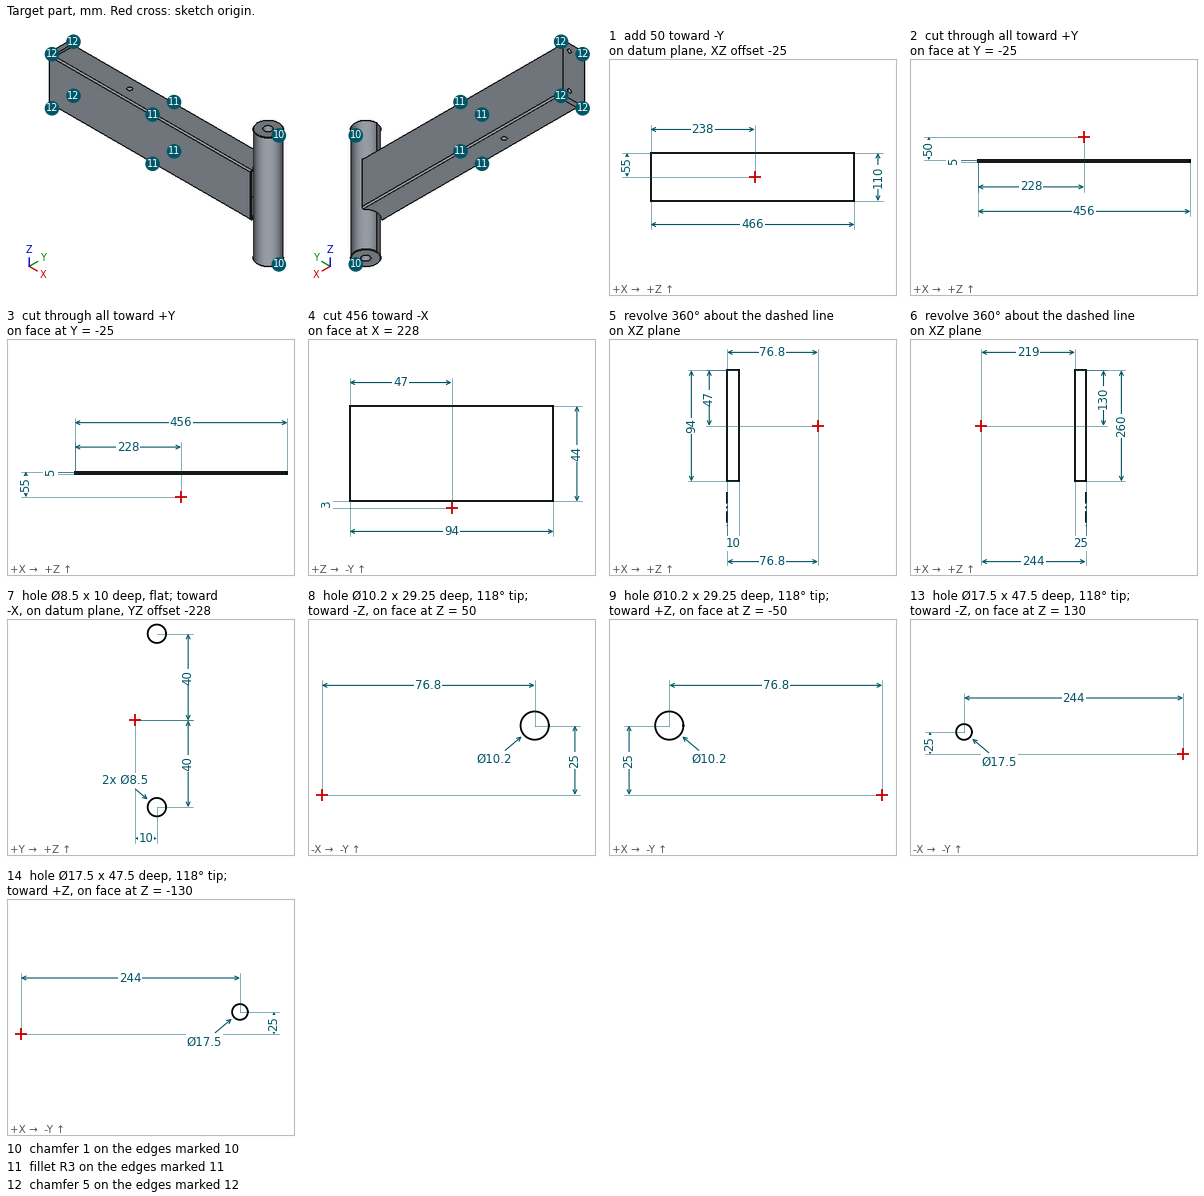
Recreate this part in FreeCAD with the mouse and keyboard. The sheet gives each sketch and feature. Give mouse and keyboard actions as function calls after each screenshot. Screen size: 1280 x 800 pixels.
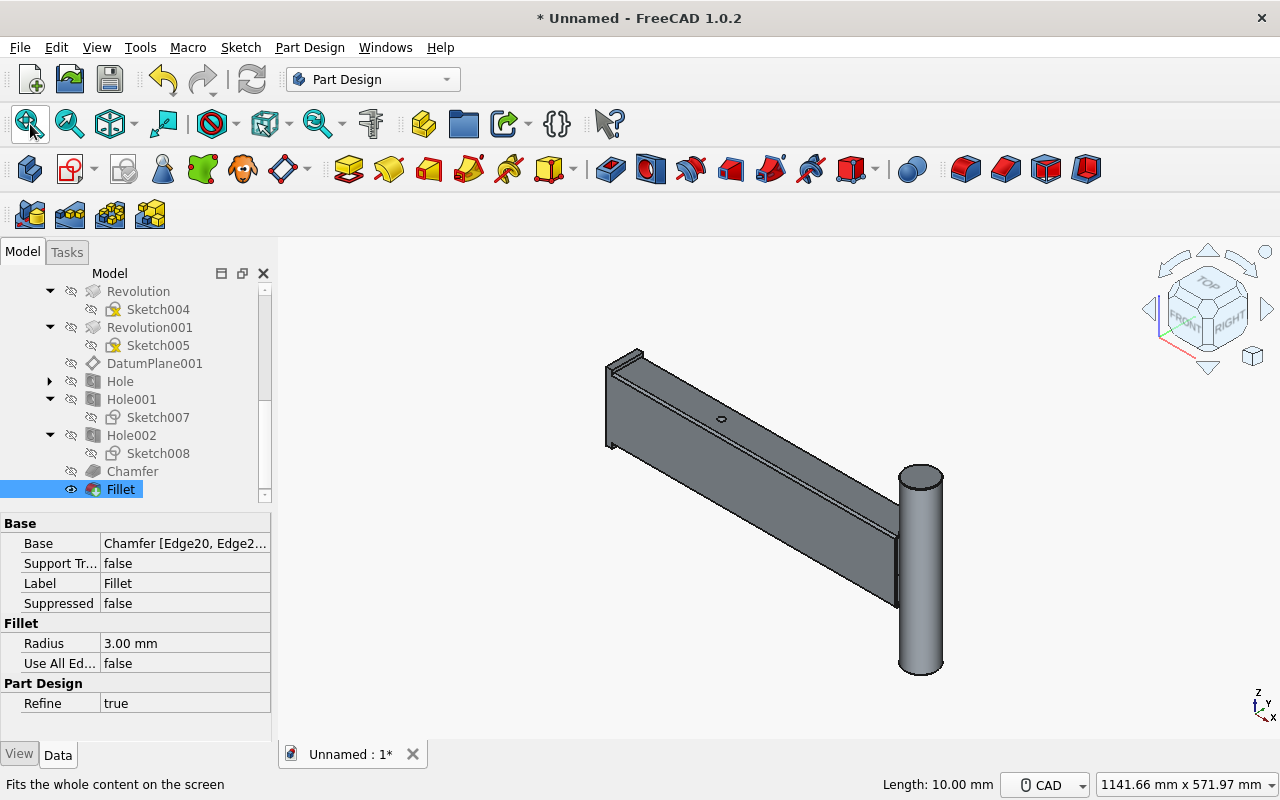
scroll(609, 446, up, 8)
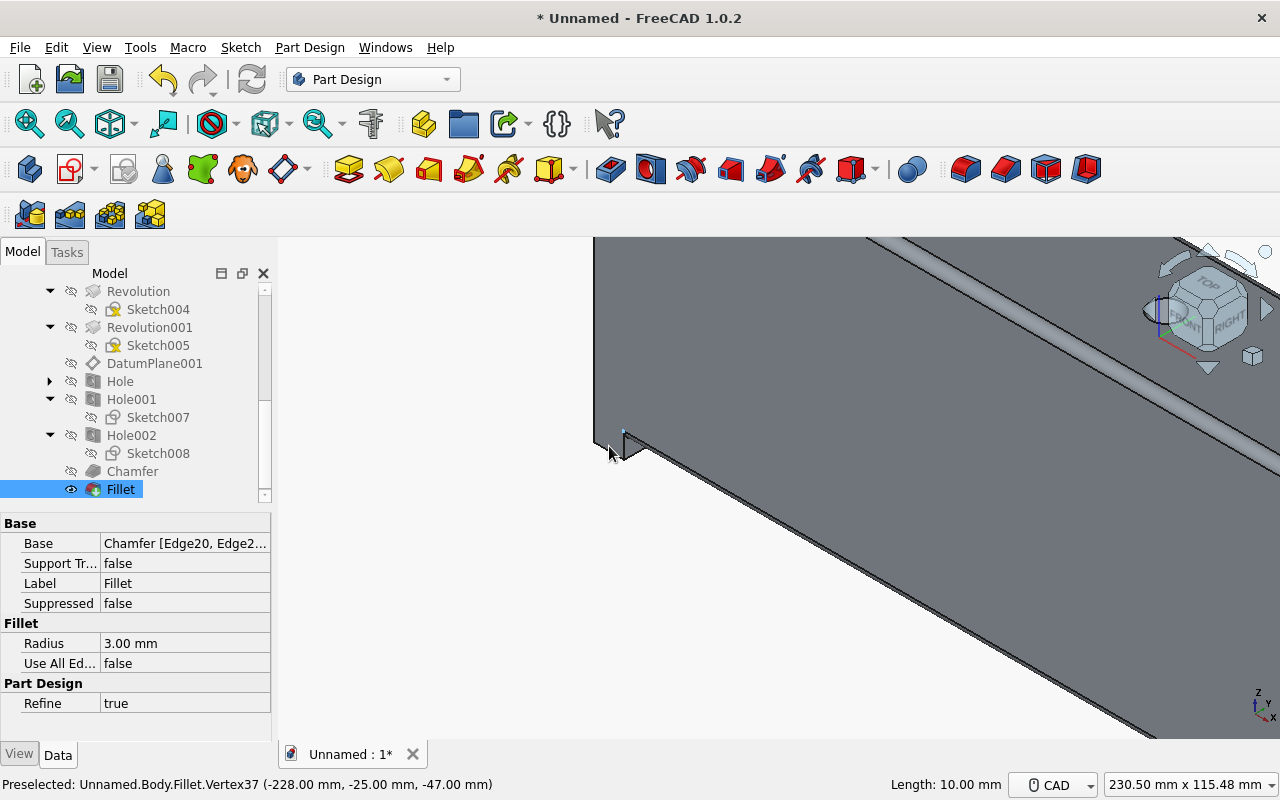
click(30, 124)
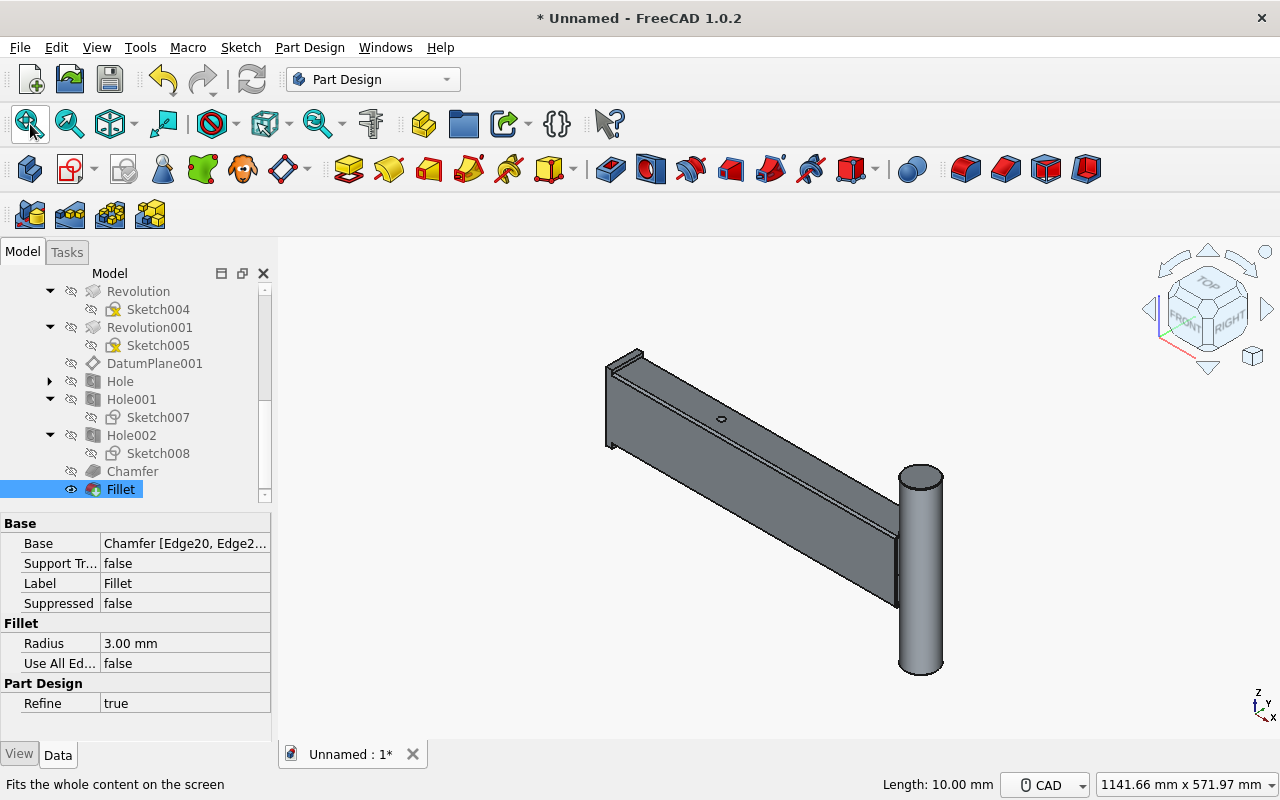
key(2)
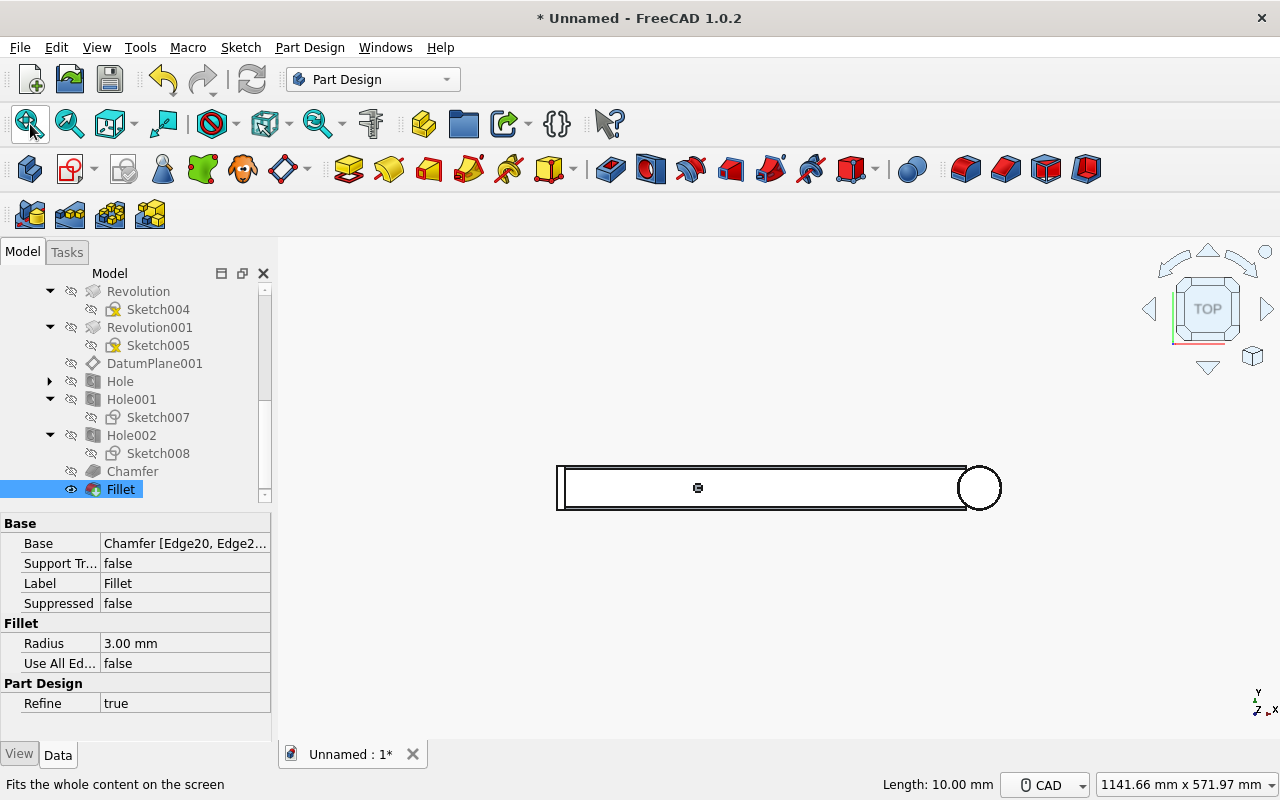
click(30, 124)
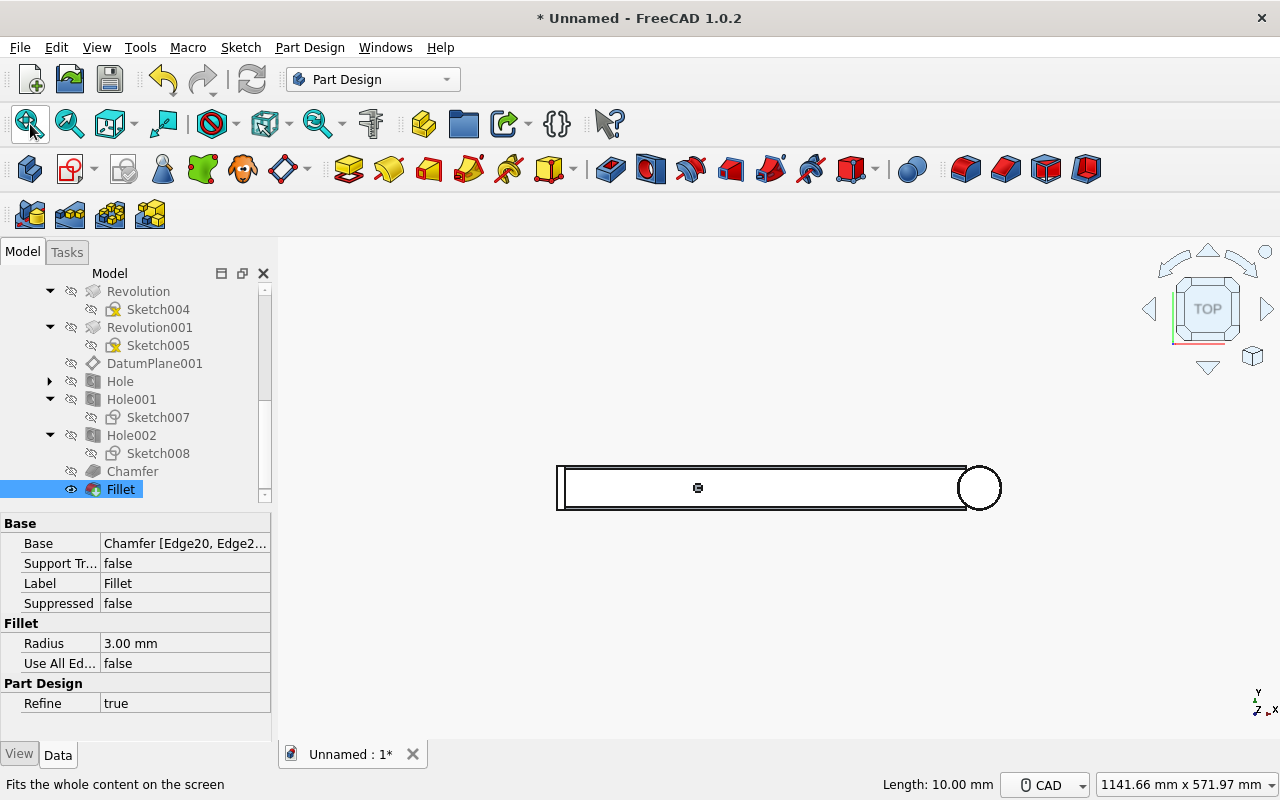
scroll(561, 509, up, 8)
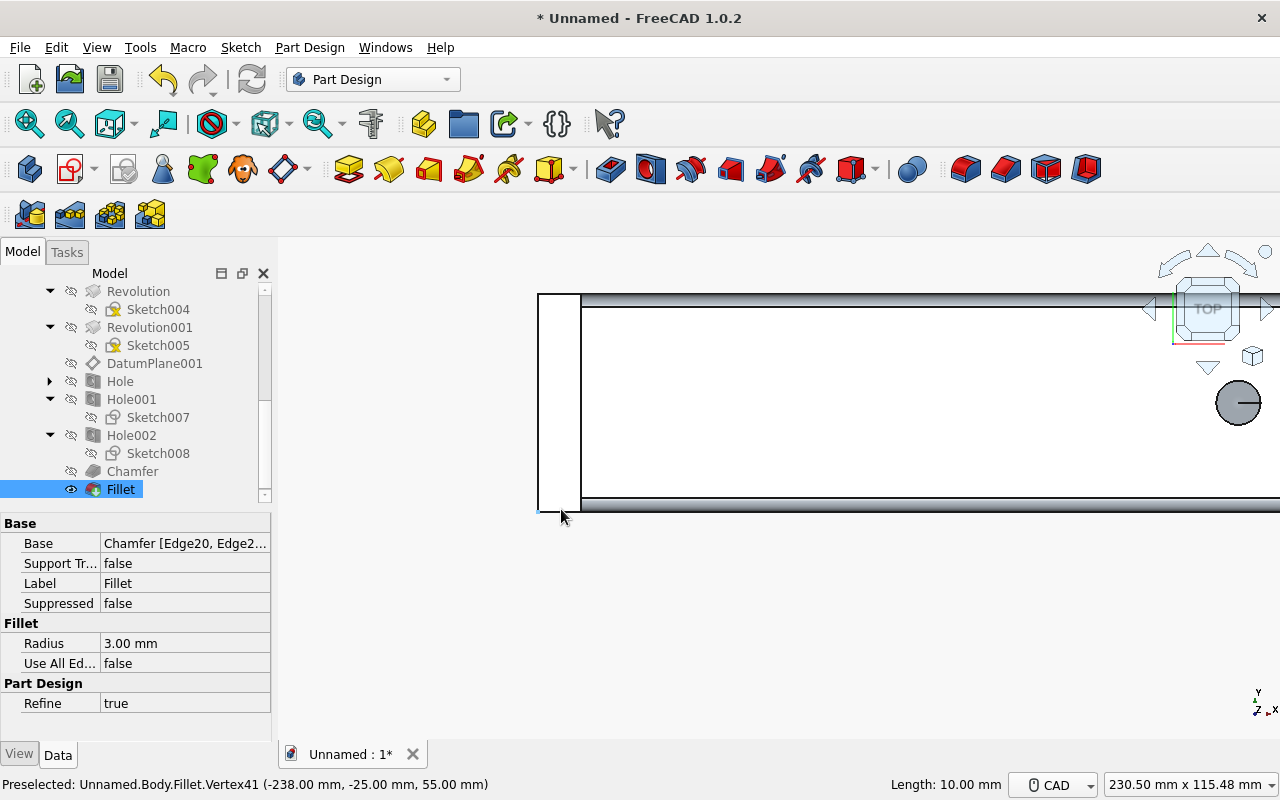
click(559, 293, ctrl)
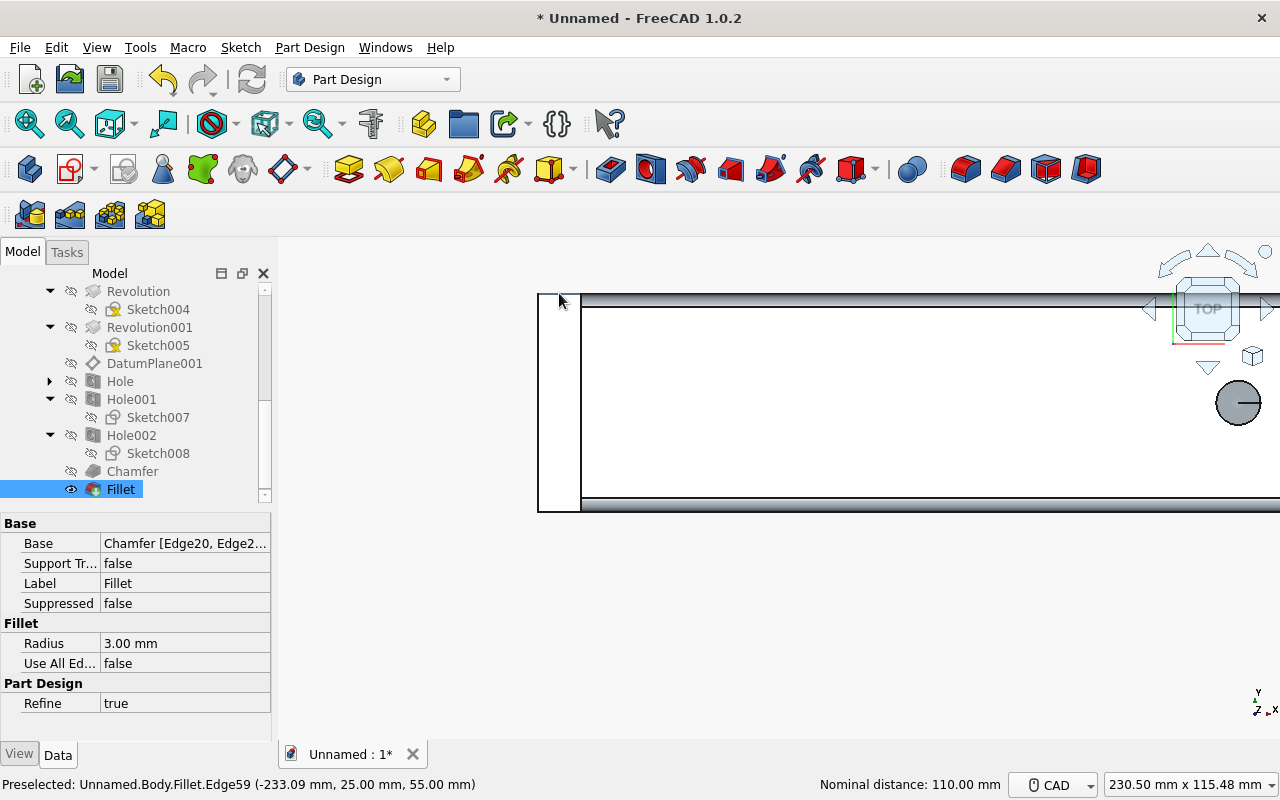
click(30, 124)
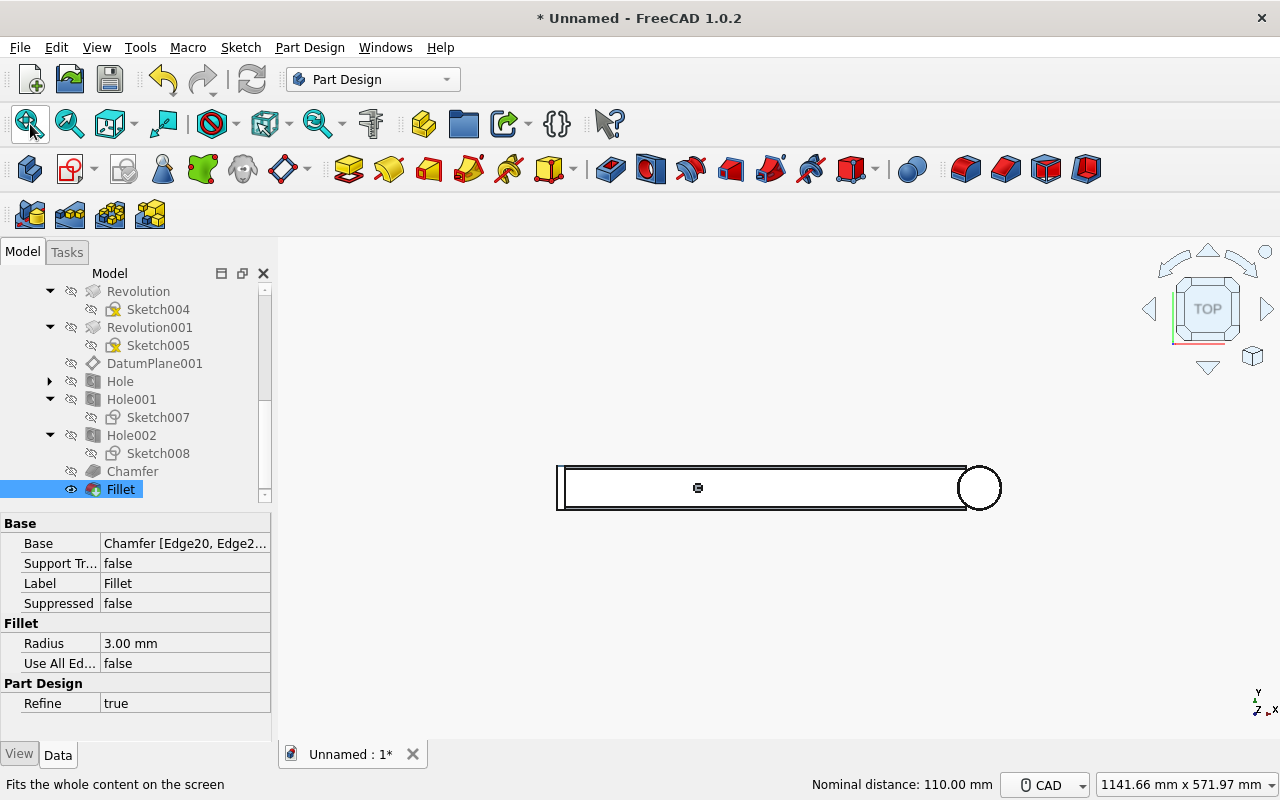
key(1)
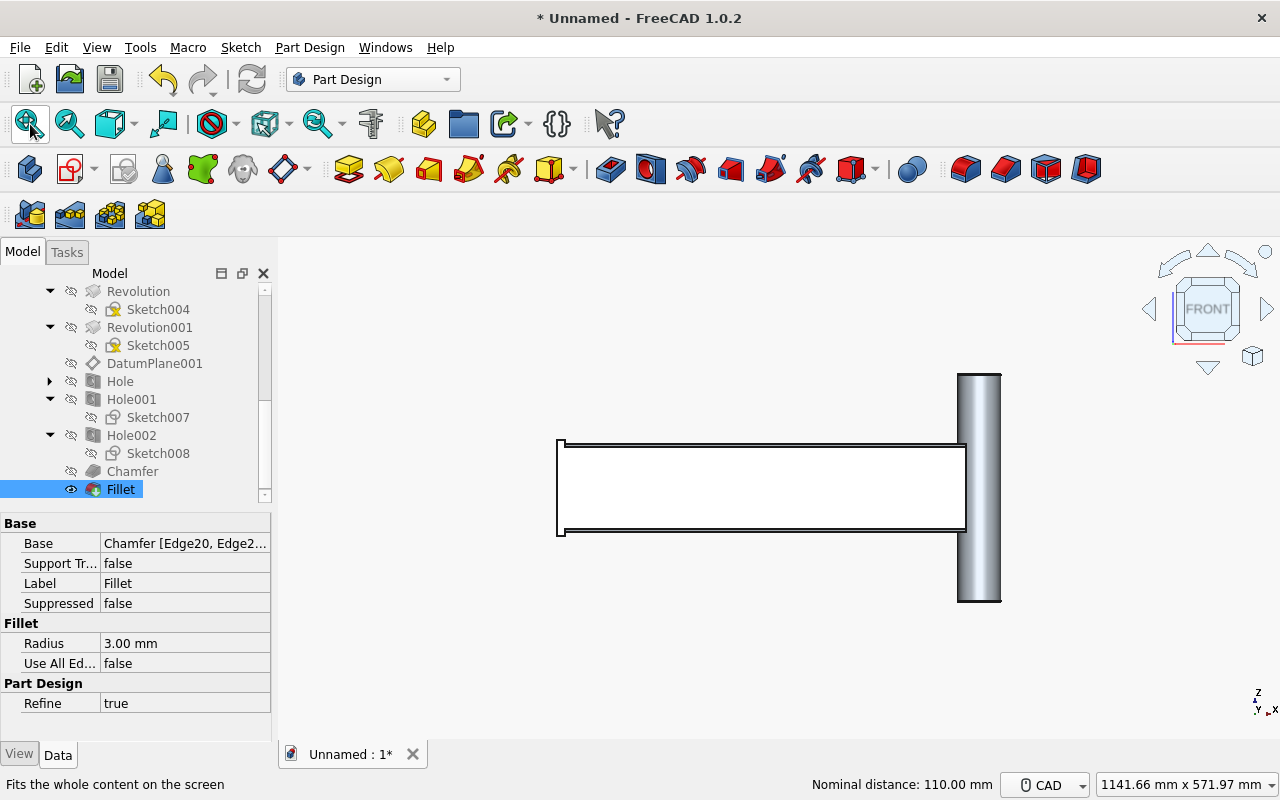
scroll(561, 535, up, 8)